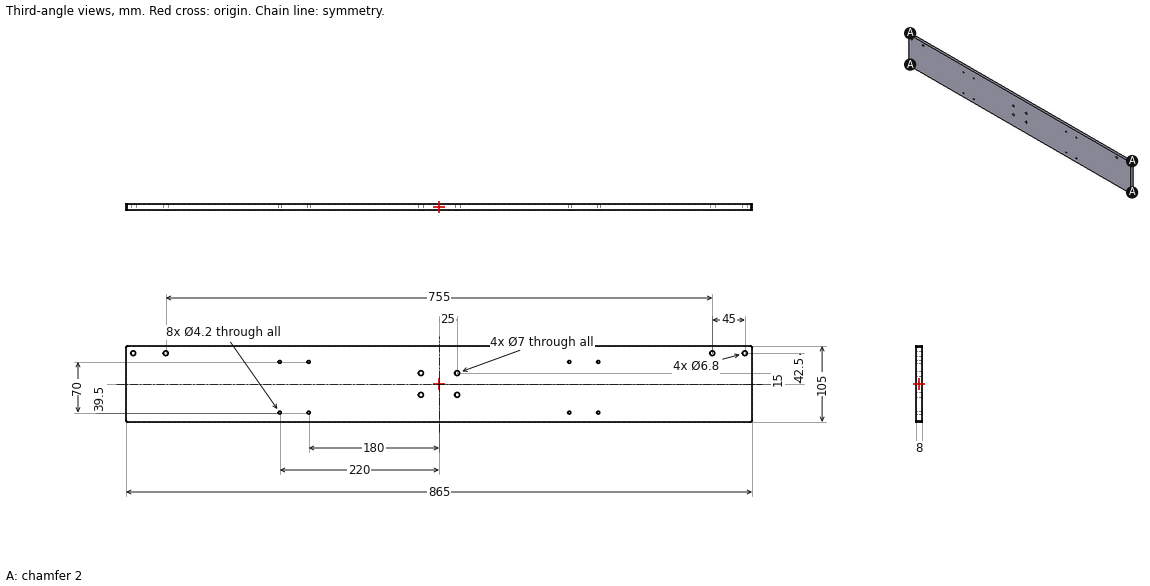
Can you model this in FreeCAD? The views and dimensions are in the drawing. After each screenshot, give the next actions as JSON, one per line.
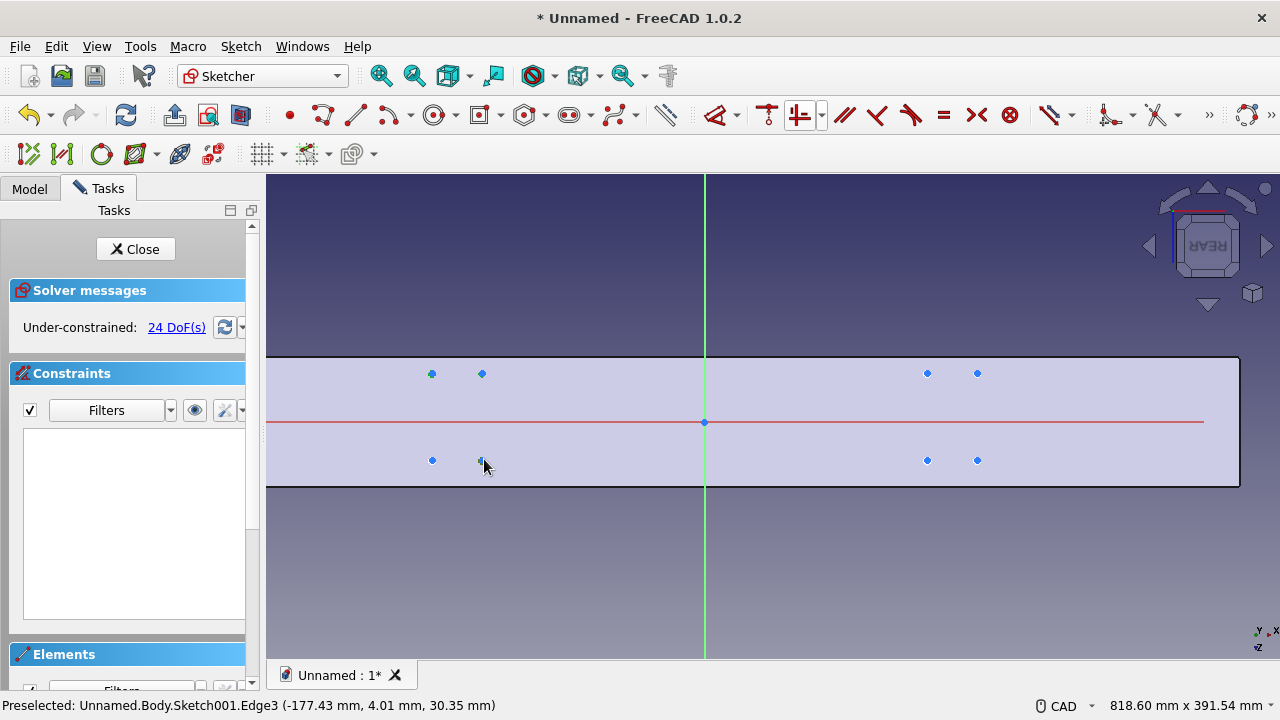
{"action": "scroll", "coordinate": [434, 459], "scroll_direction": "up", "scroll_amount": 8}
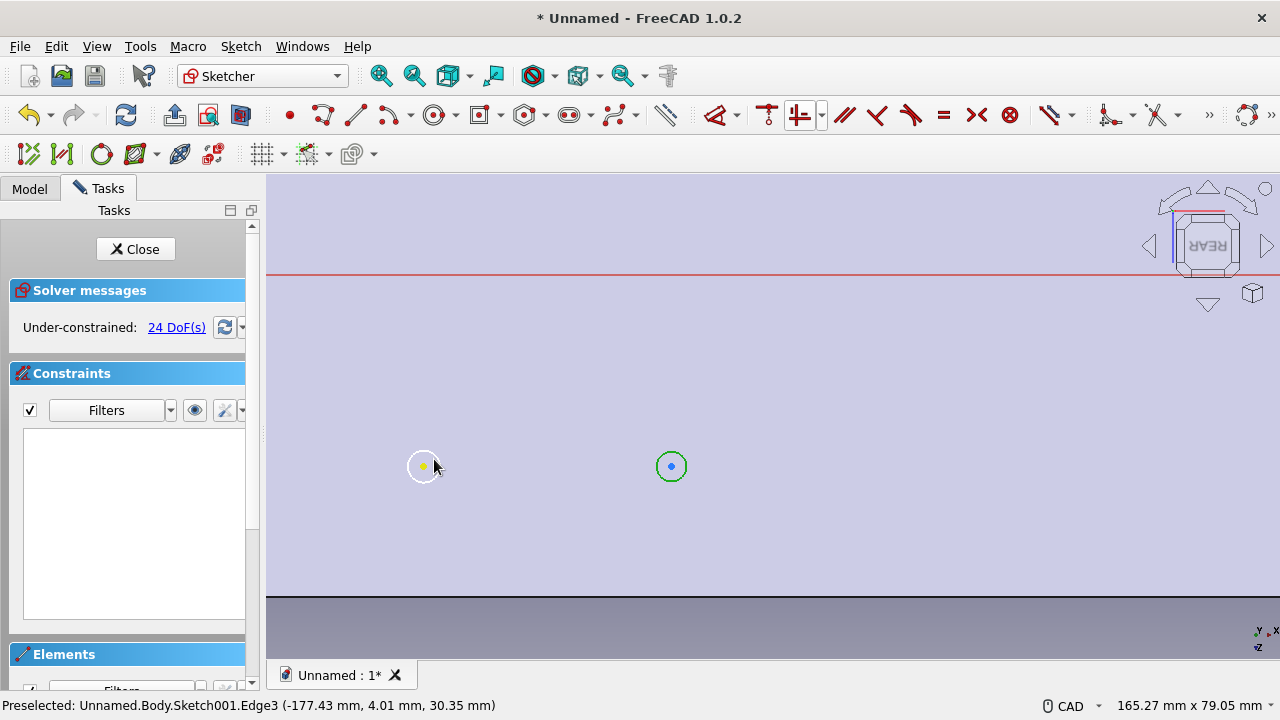
{"action": "left_click", "coordinate": [435, 455]}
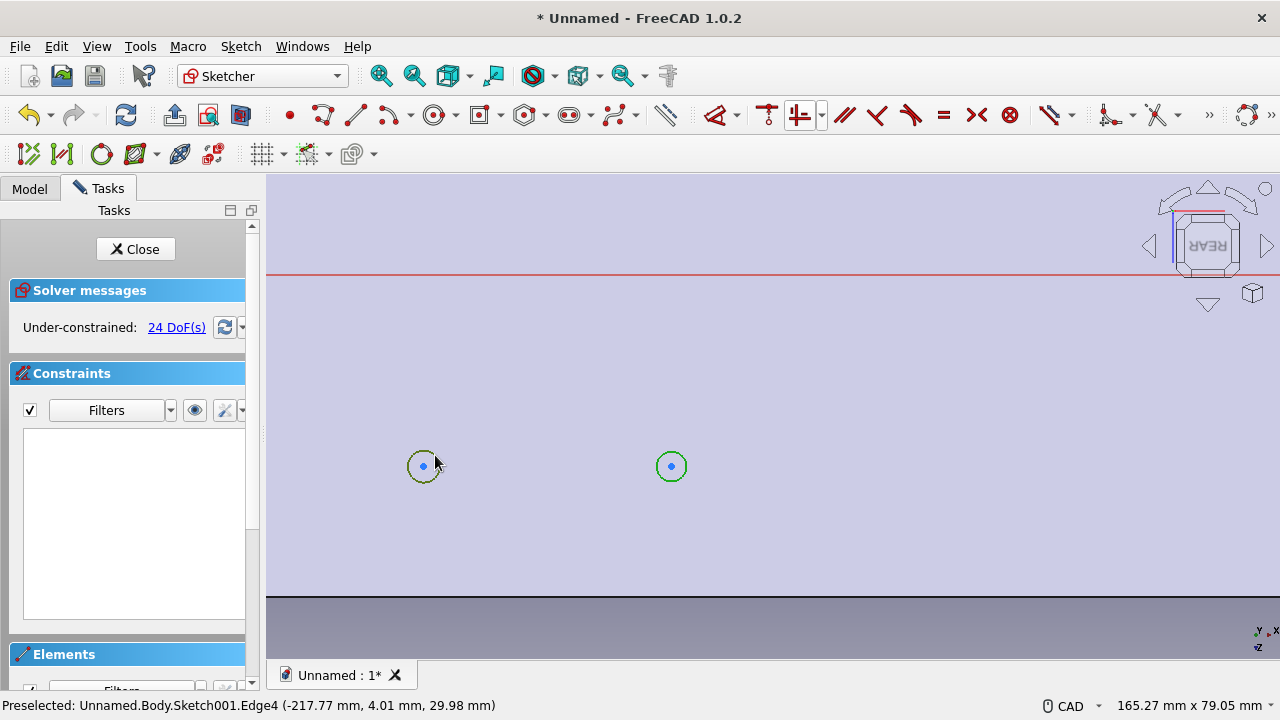
{"action": "scroll", "coordinate": [434, 459], "scroll_direction": "down", "scroll_amount": 8}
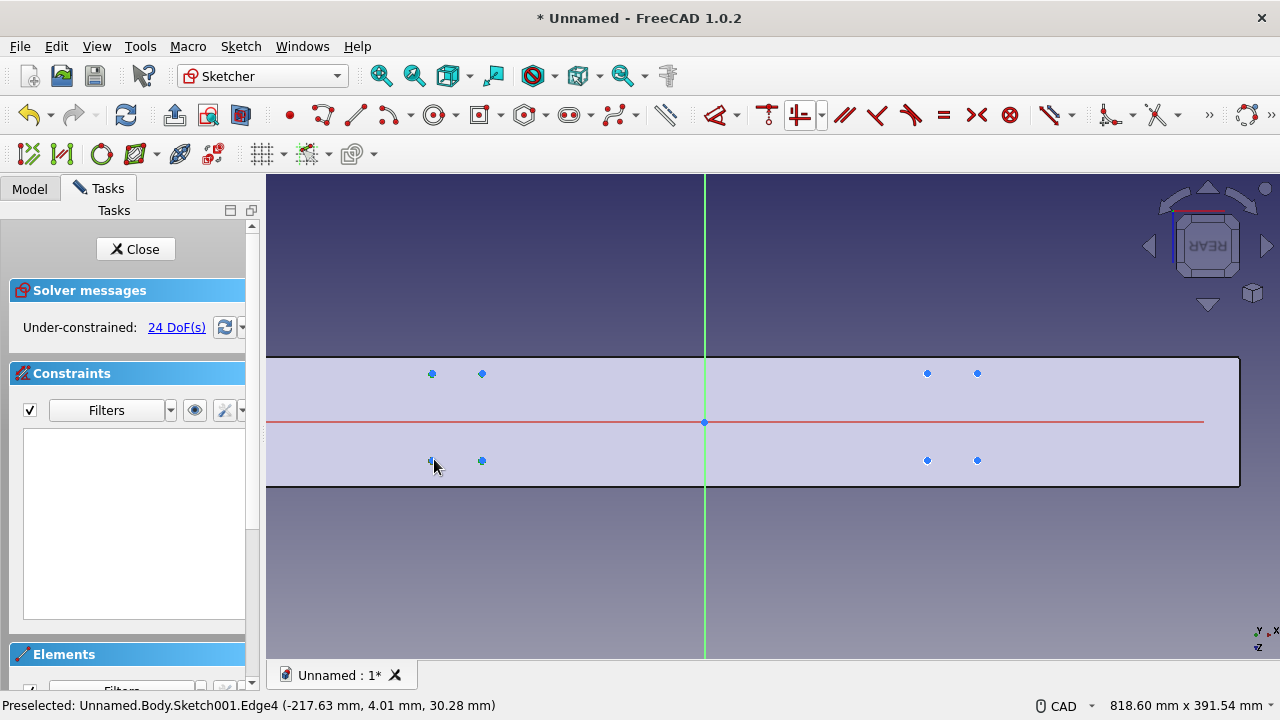
{"action": "scroll", "coordinate": [979, 459], "scroll_direction": "up", "scroll_amount": 8}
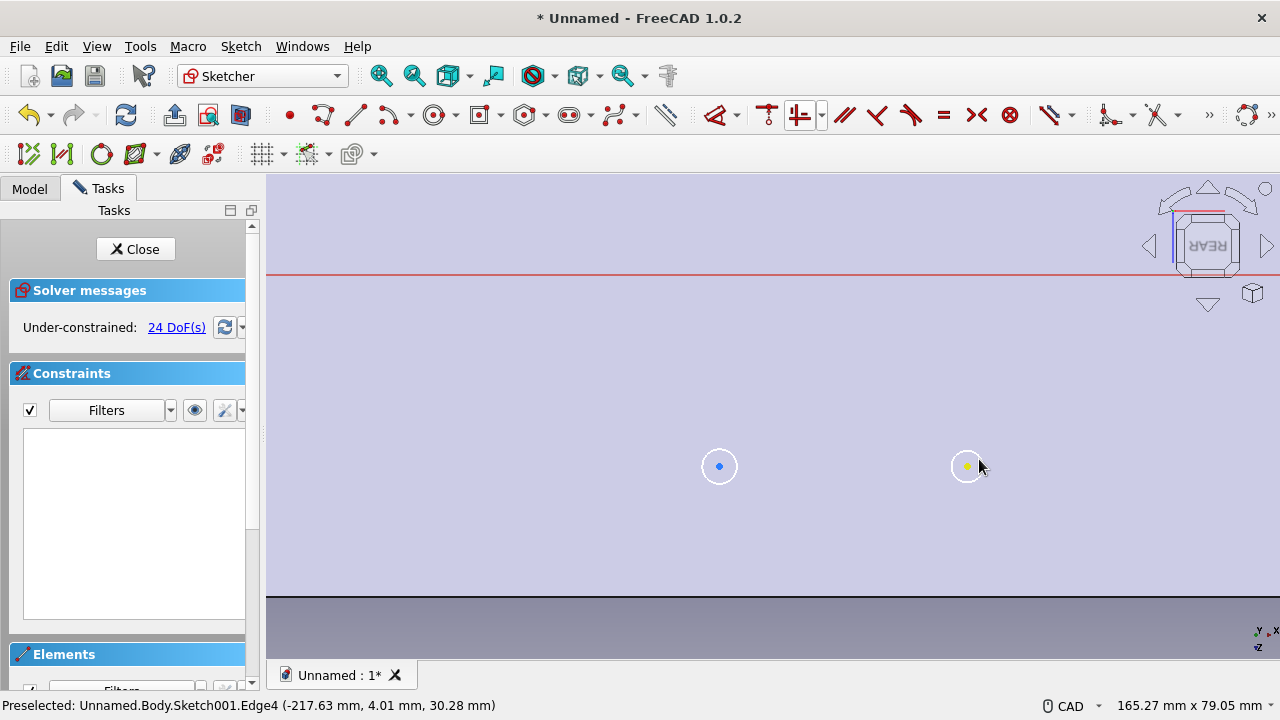
{"action": "left_click", "coordinate": [978, 455]}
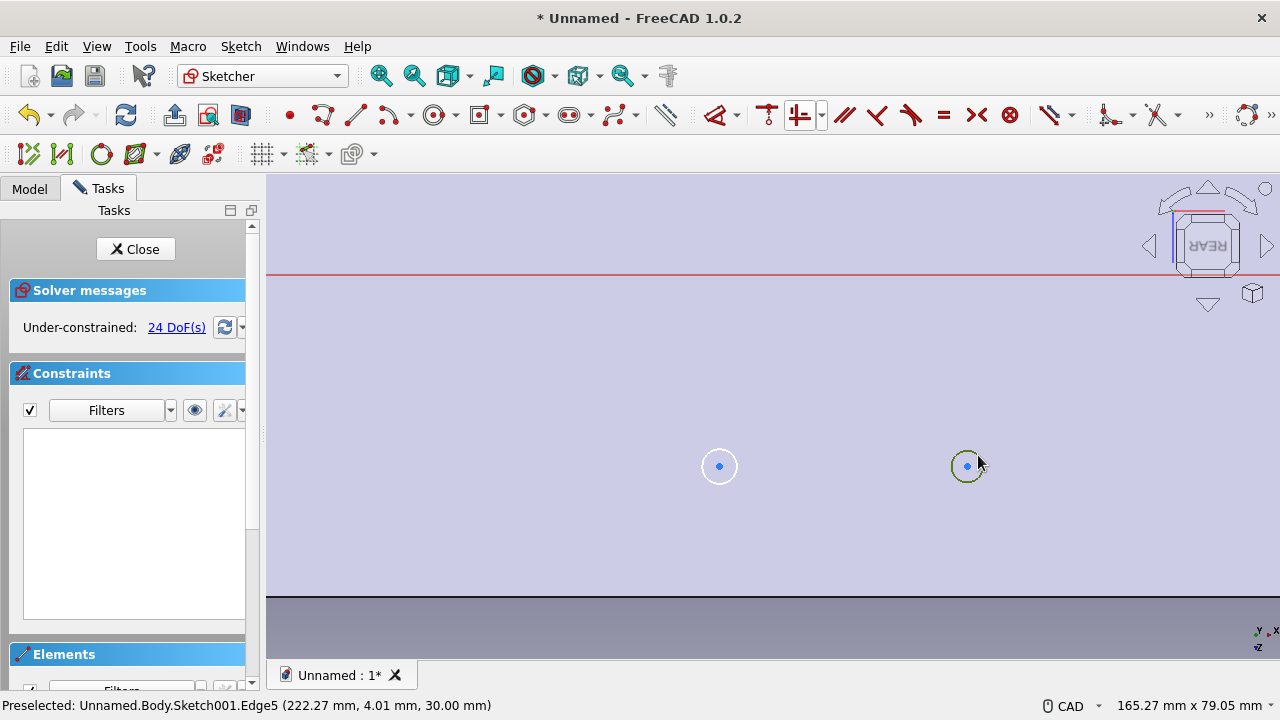
{"action": "left_click", "coordinate": [732, 454]}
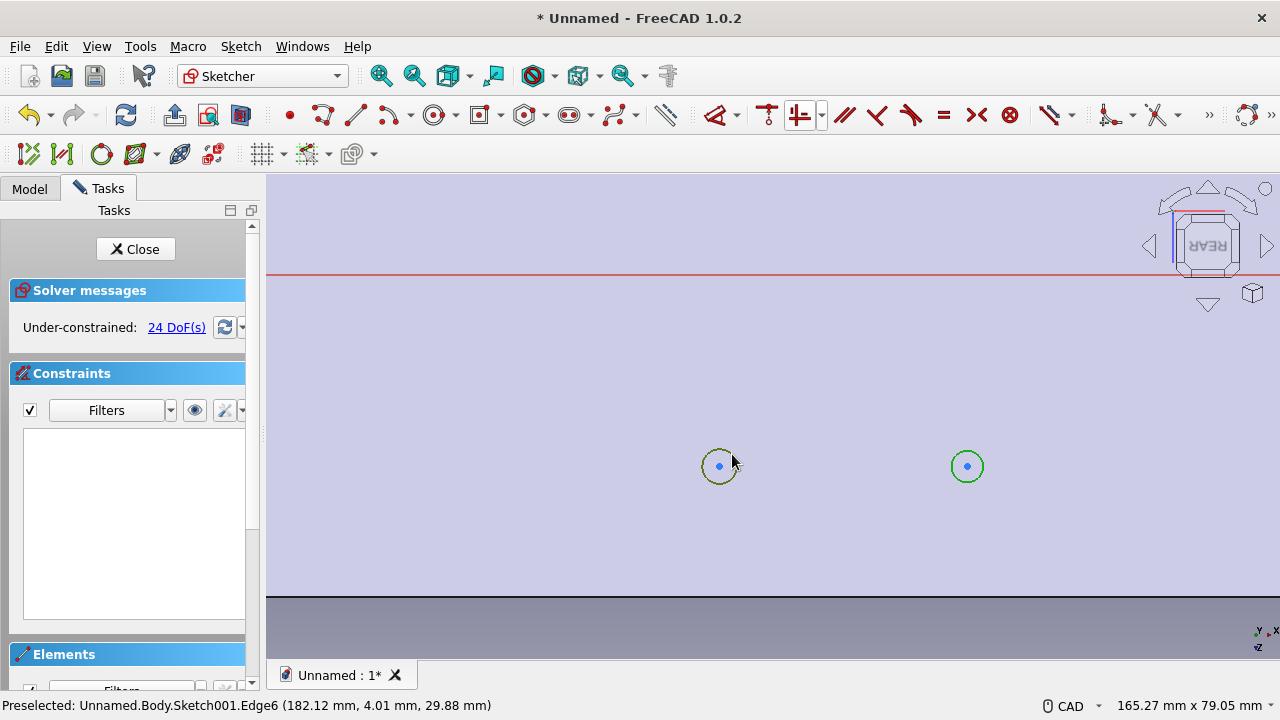
{"action": "scroll", "coordinate": [979, 459], "scroll_direction": "down", "scroll_amount": 8}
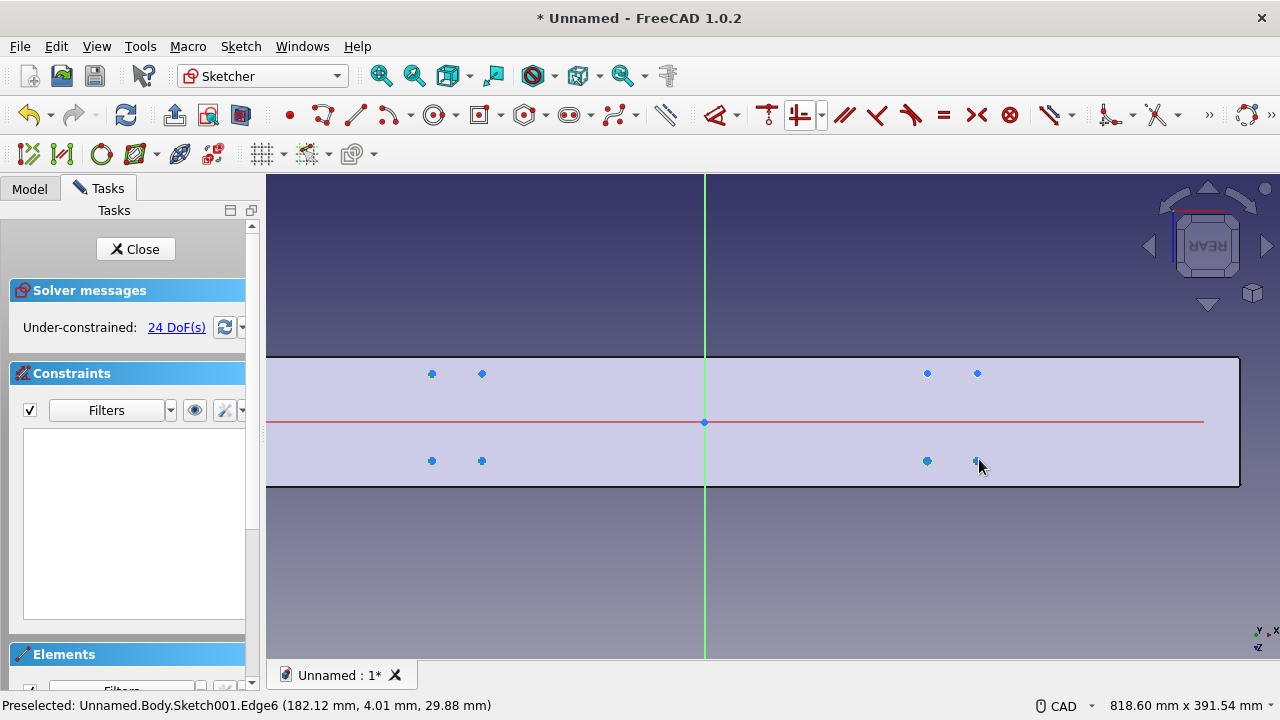
{"action": "scroll", "coordinate": [930, 372], "scroll_direction": "up", "scroll_amount": 8}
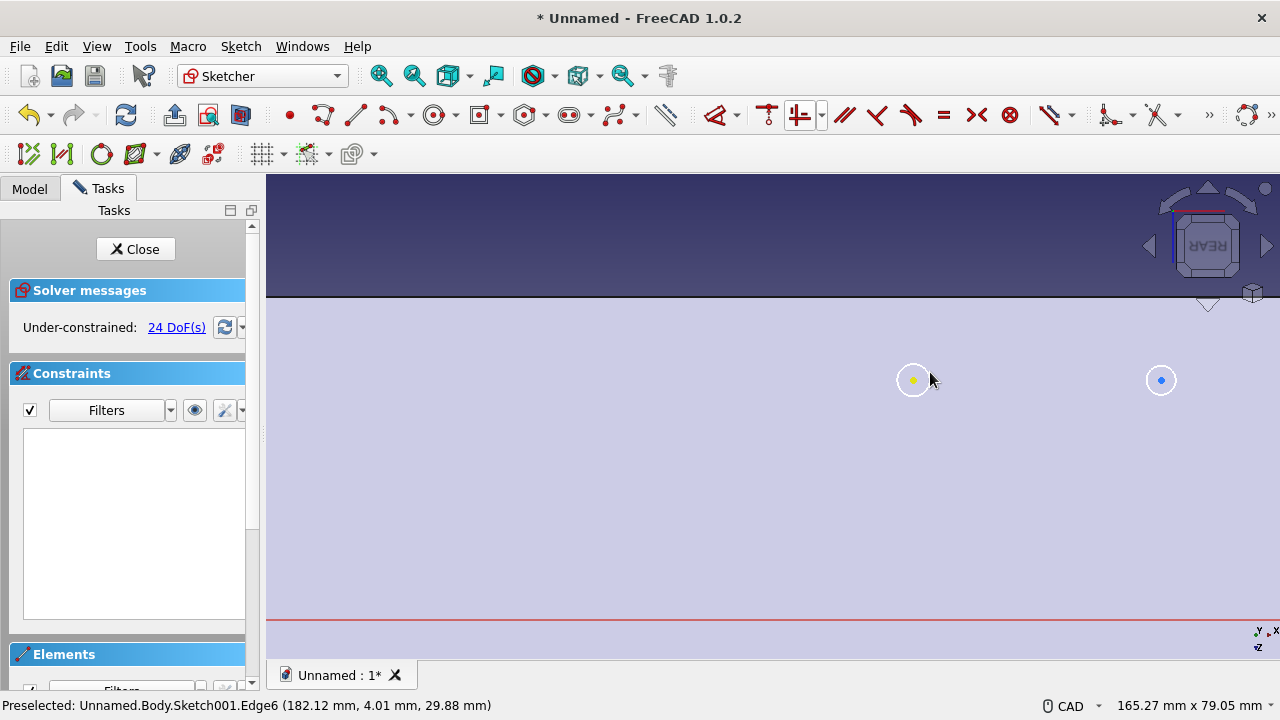
{"action": "left_click", "coordinate": [925, 369]}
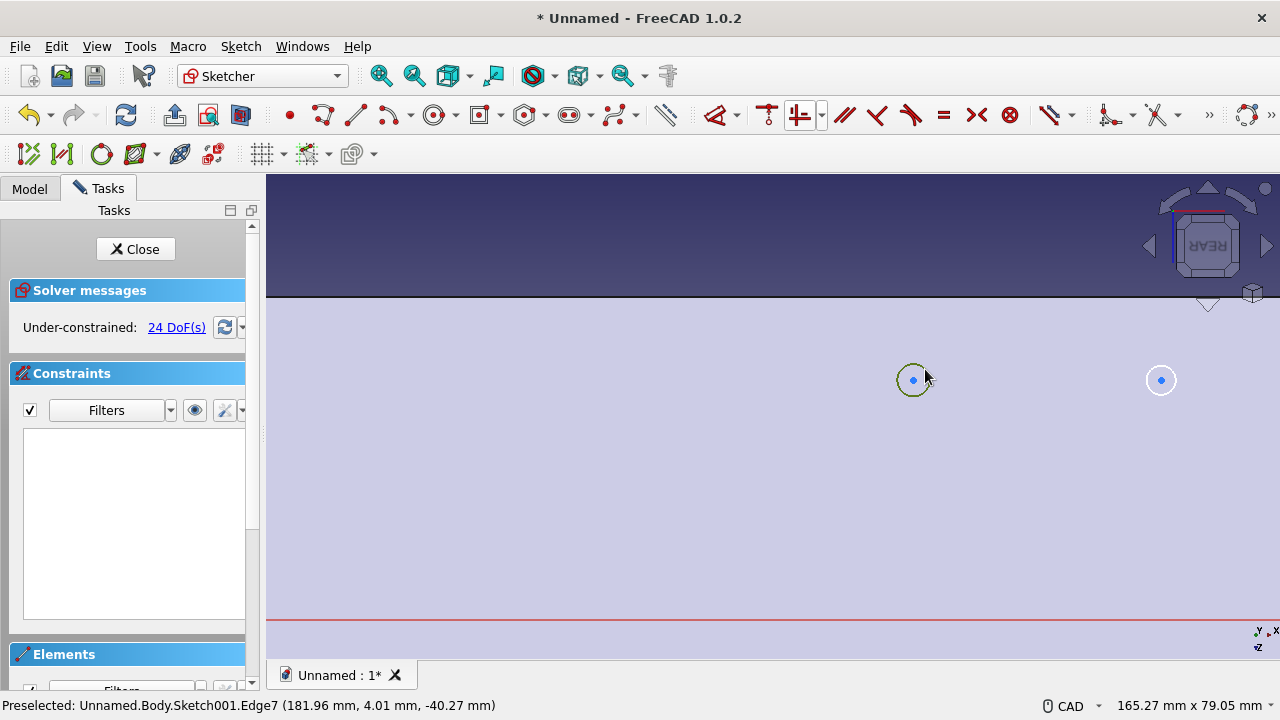
{"action": "scroll", "coordinate": [930, 372], "scroll_direction": "down", "scroll_amount": 8}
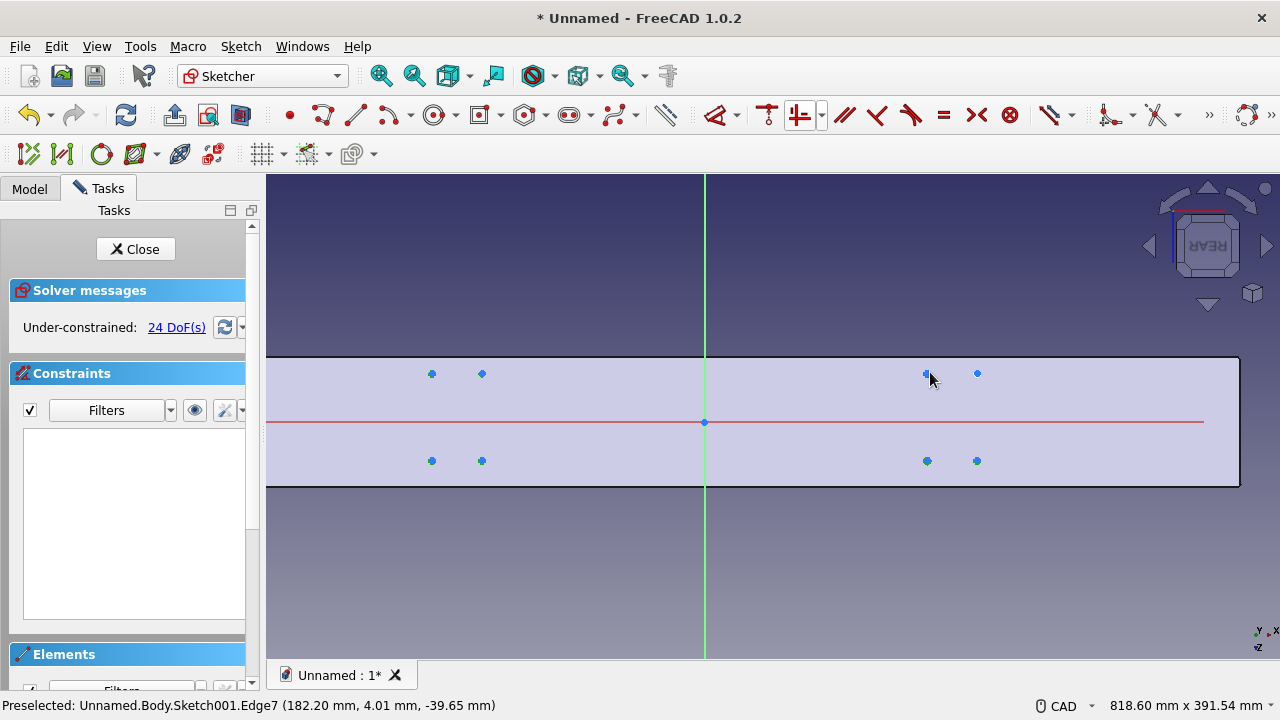
{"action": "scroll", "coordinate": [979, 372], "scroll_direction": "up", "scroll_amount": 8}